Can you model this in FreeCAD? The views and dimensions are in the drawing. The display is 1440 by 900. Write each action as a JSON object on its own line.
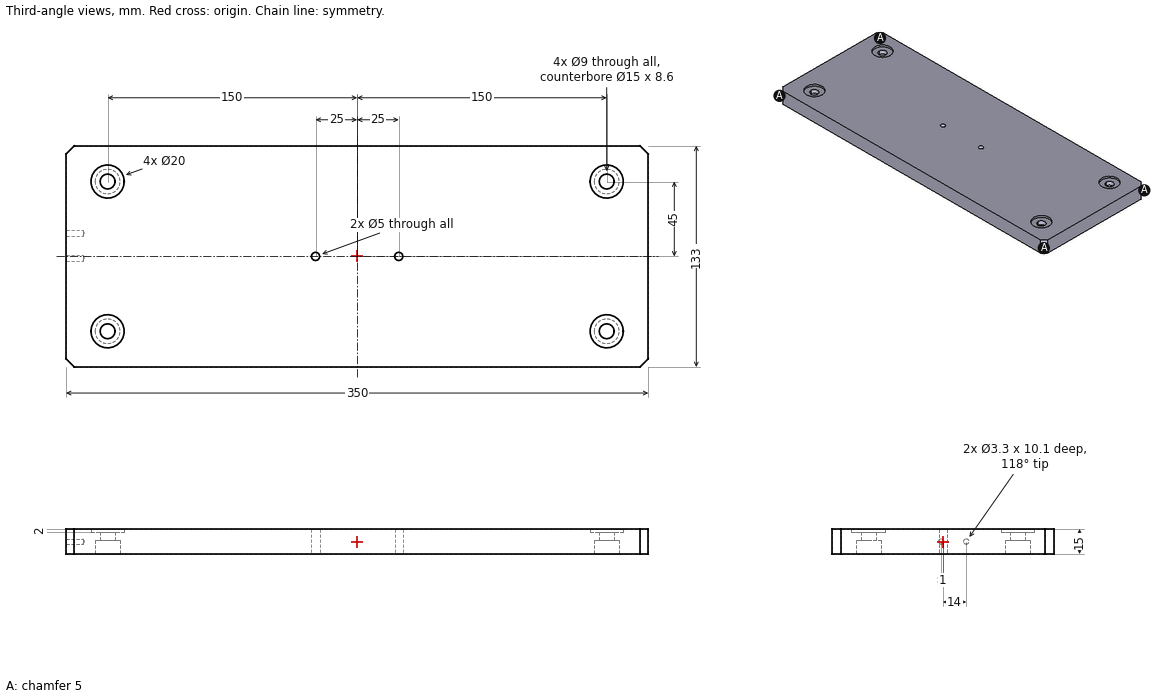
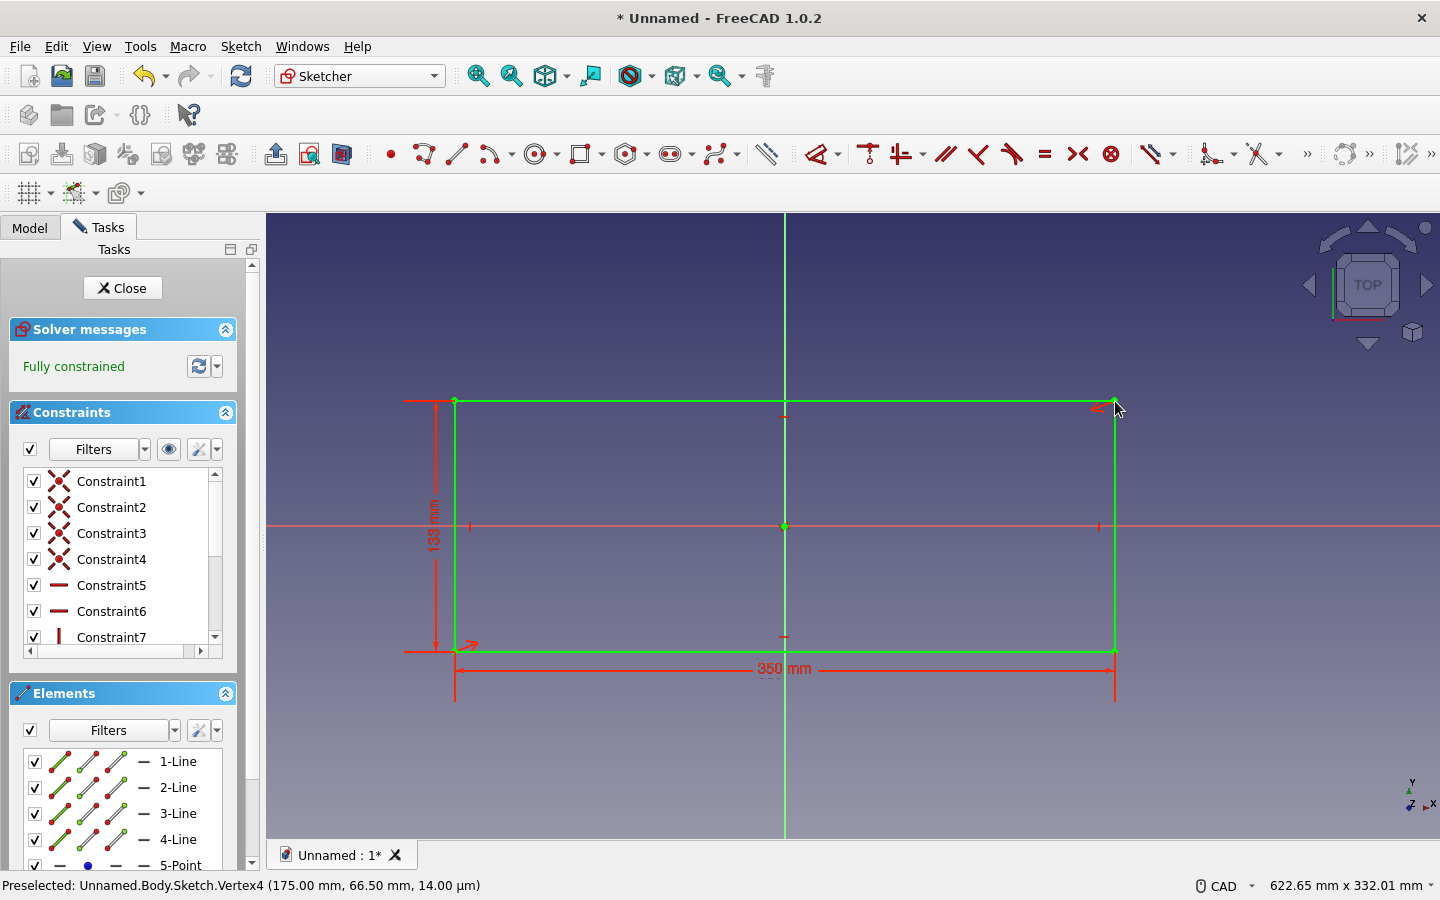
{"action": "left_click", "coordinate": [123, 288]}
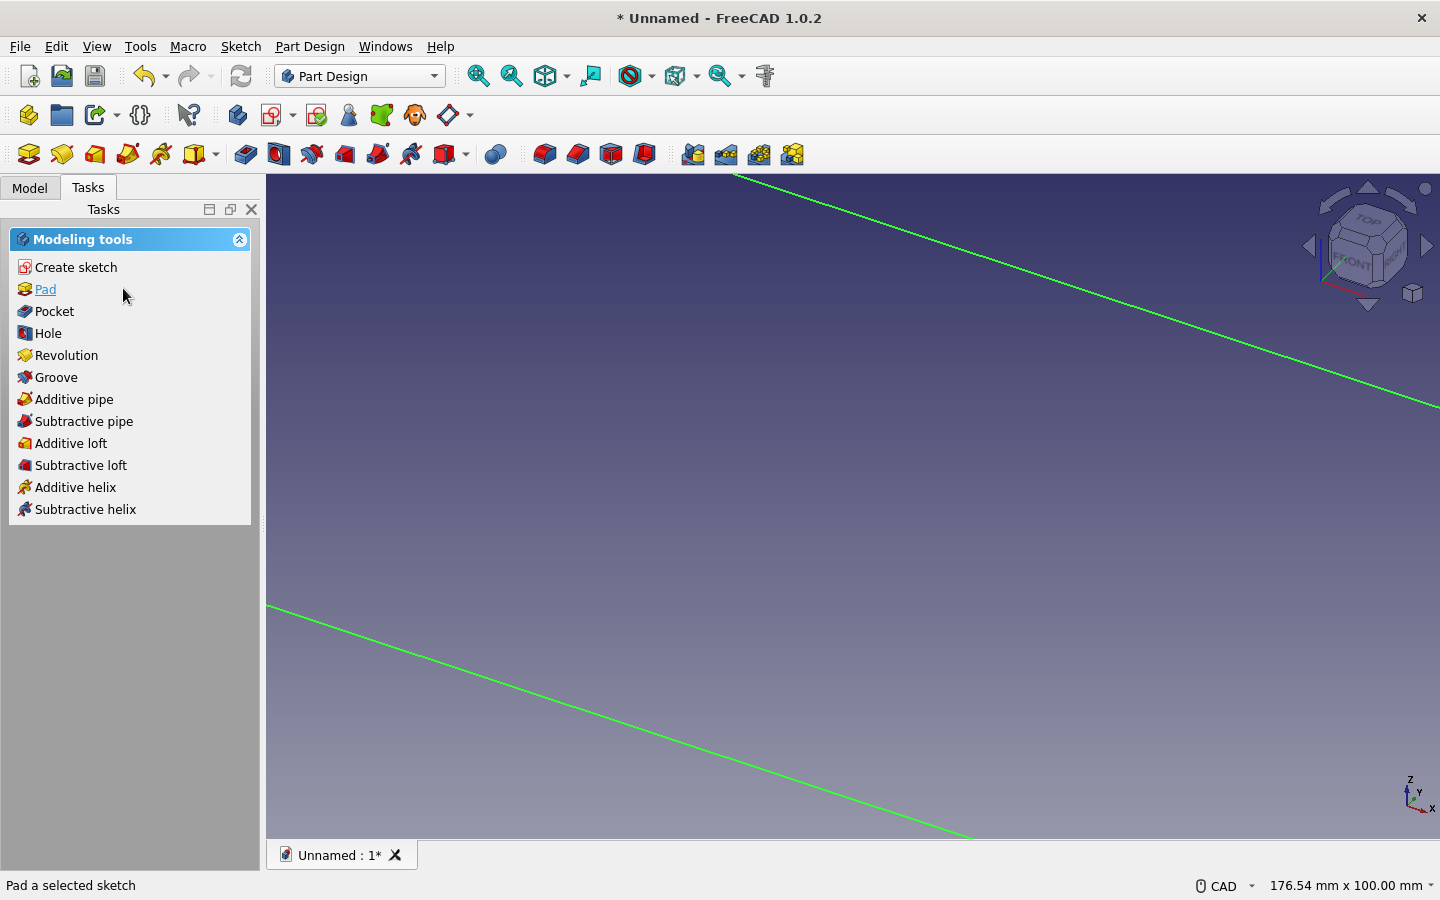
{"action": "left_click", "coordinate": [29, 154]}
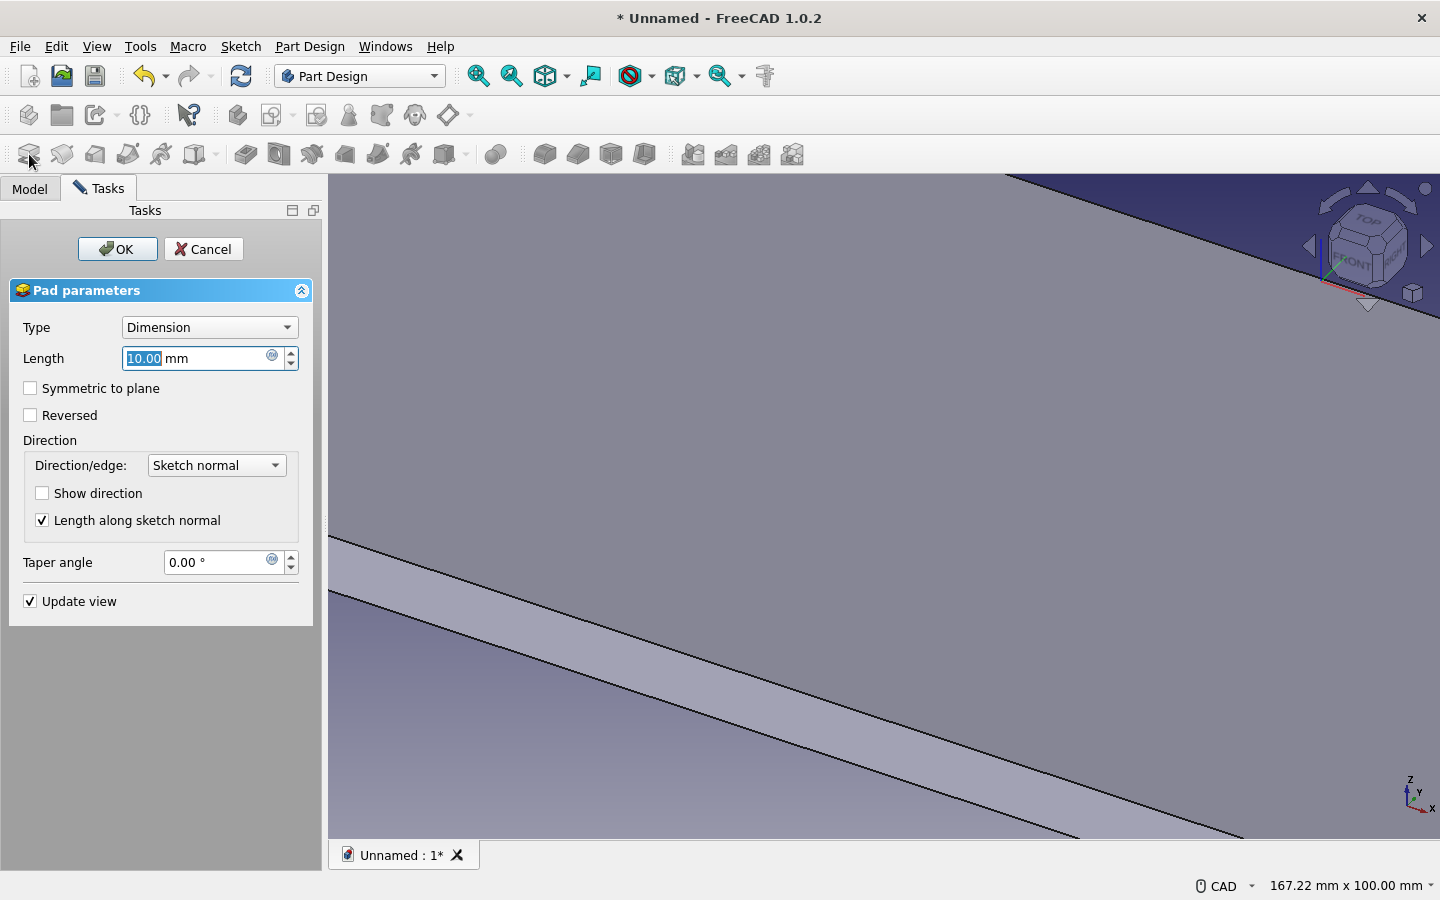
{"action": "type", "text": "15"}
{"action": "key", "text": "Tab"}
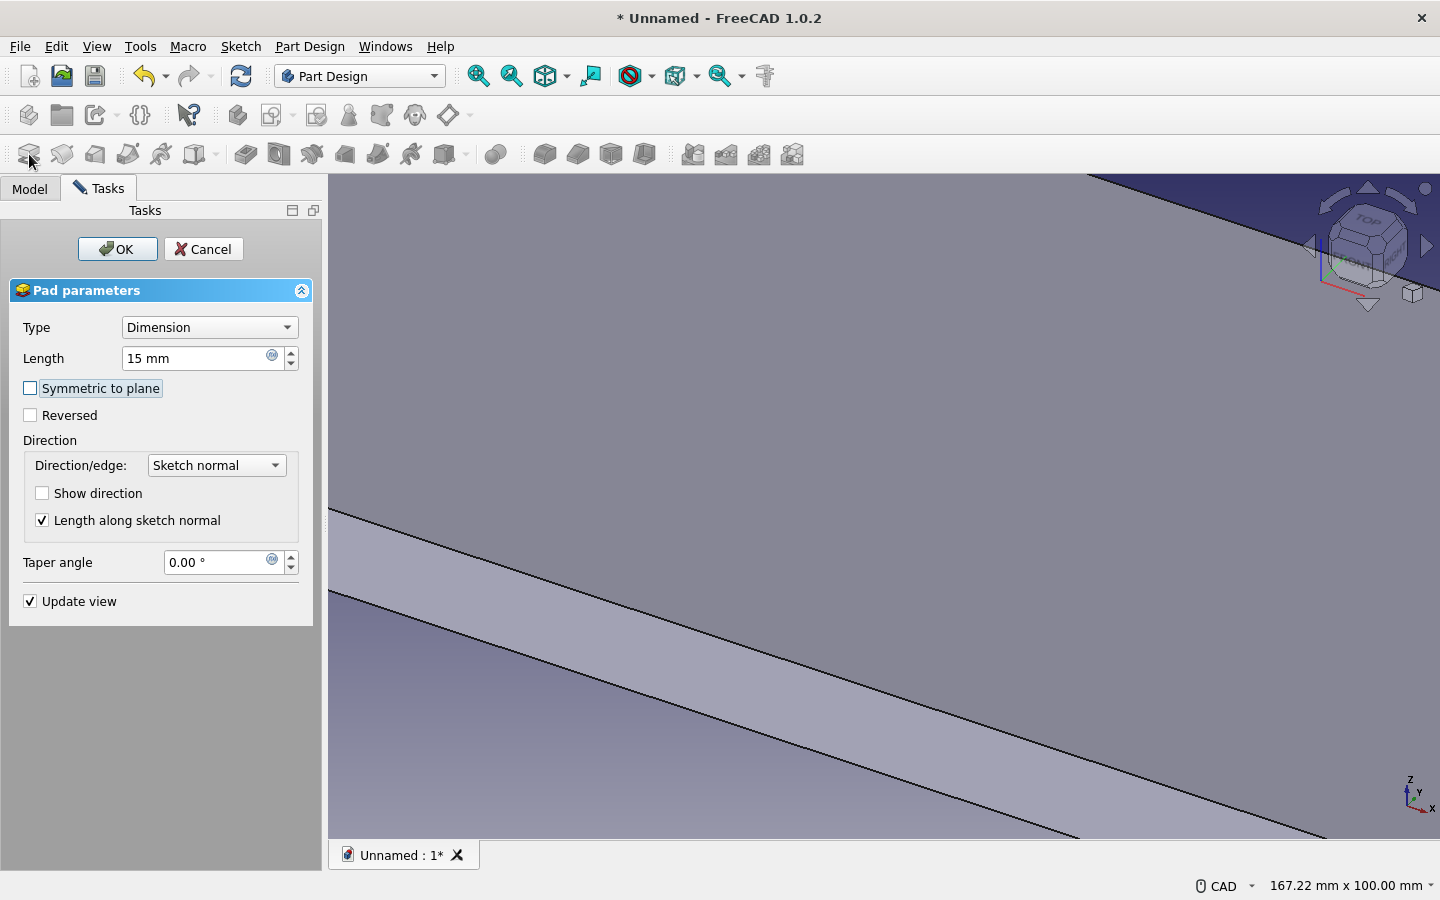
{"action": "left_click", "coordinate": [31, 388]}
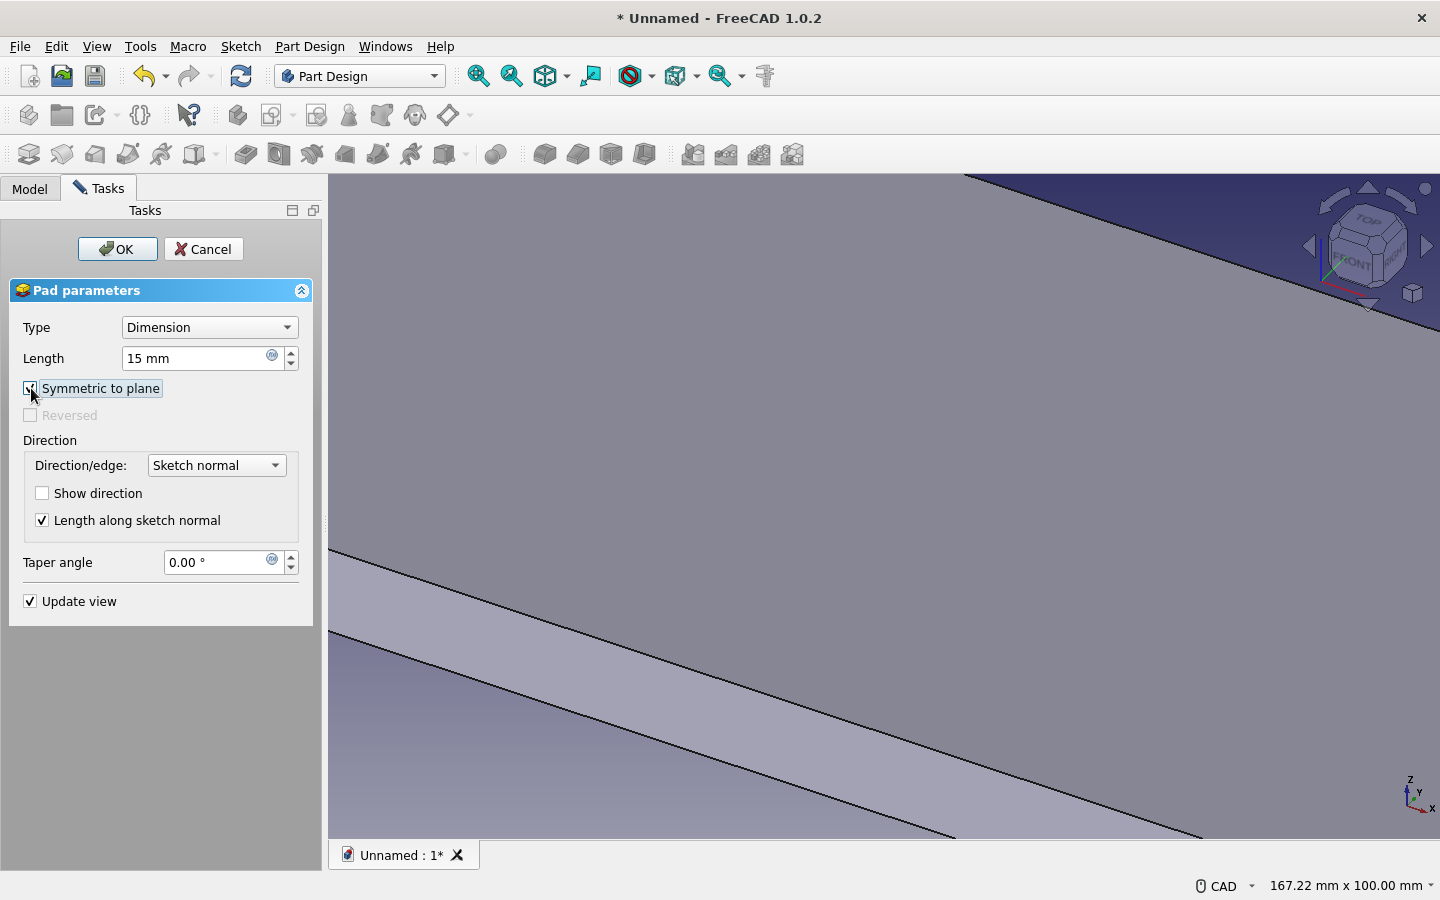
{"action": "left_click", "coordinate": [118, 249]}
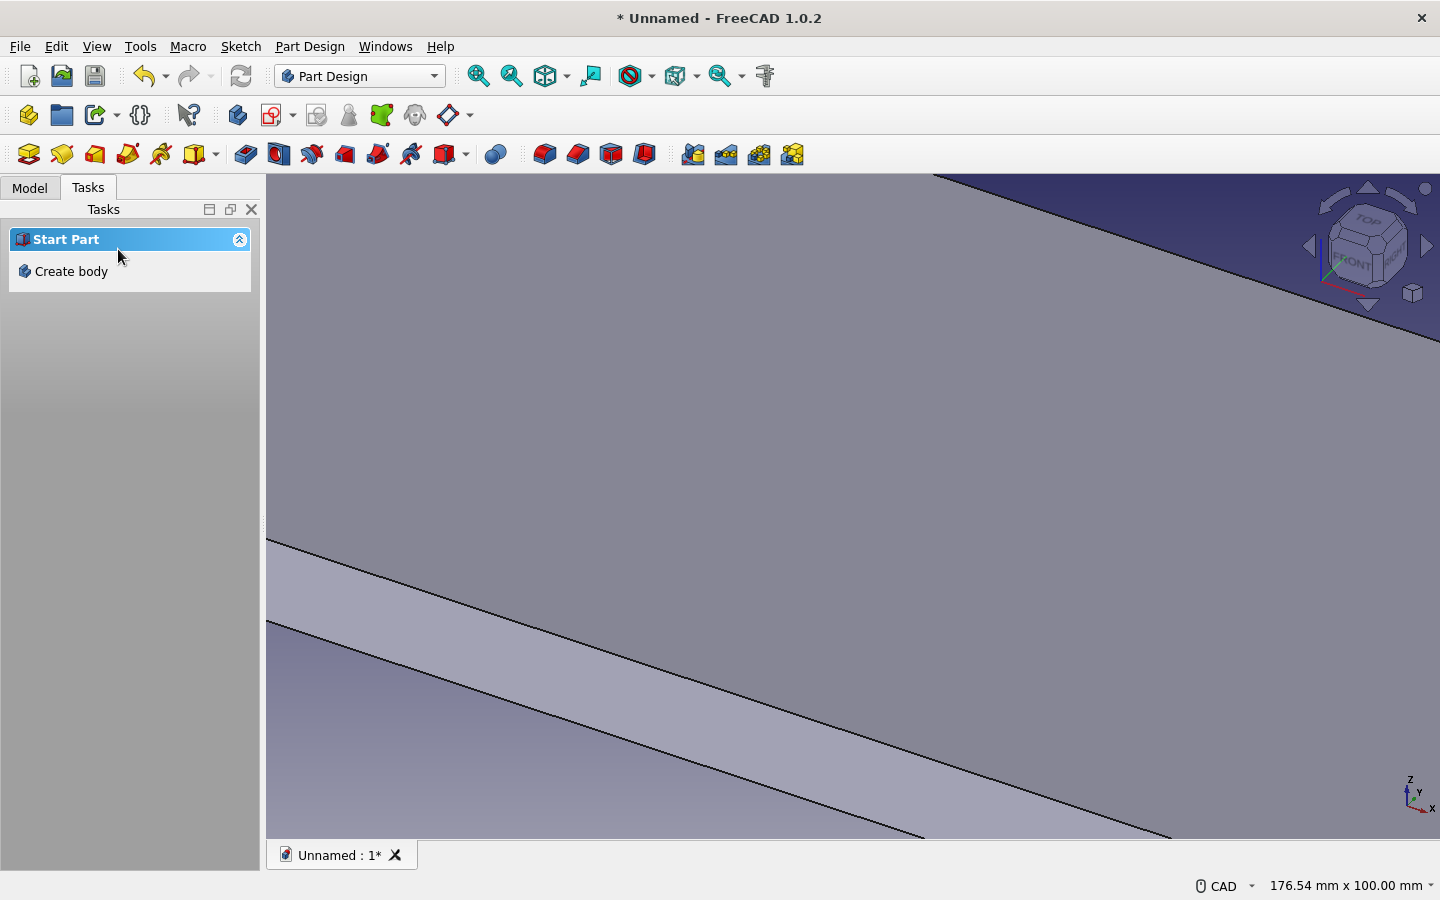
{"action": "left_click", "coordinate": [479, 76]}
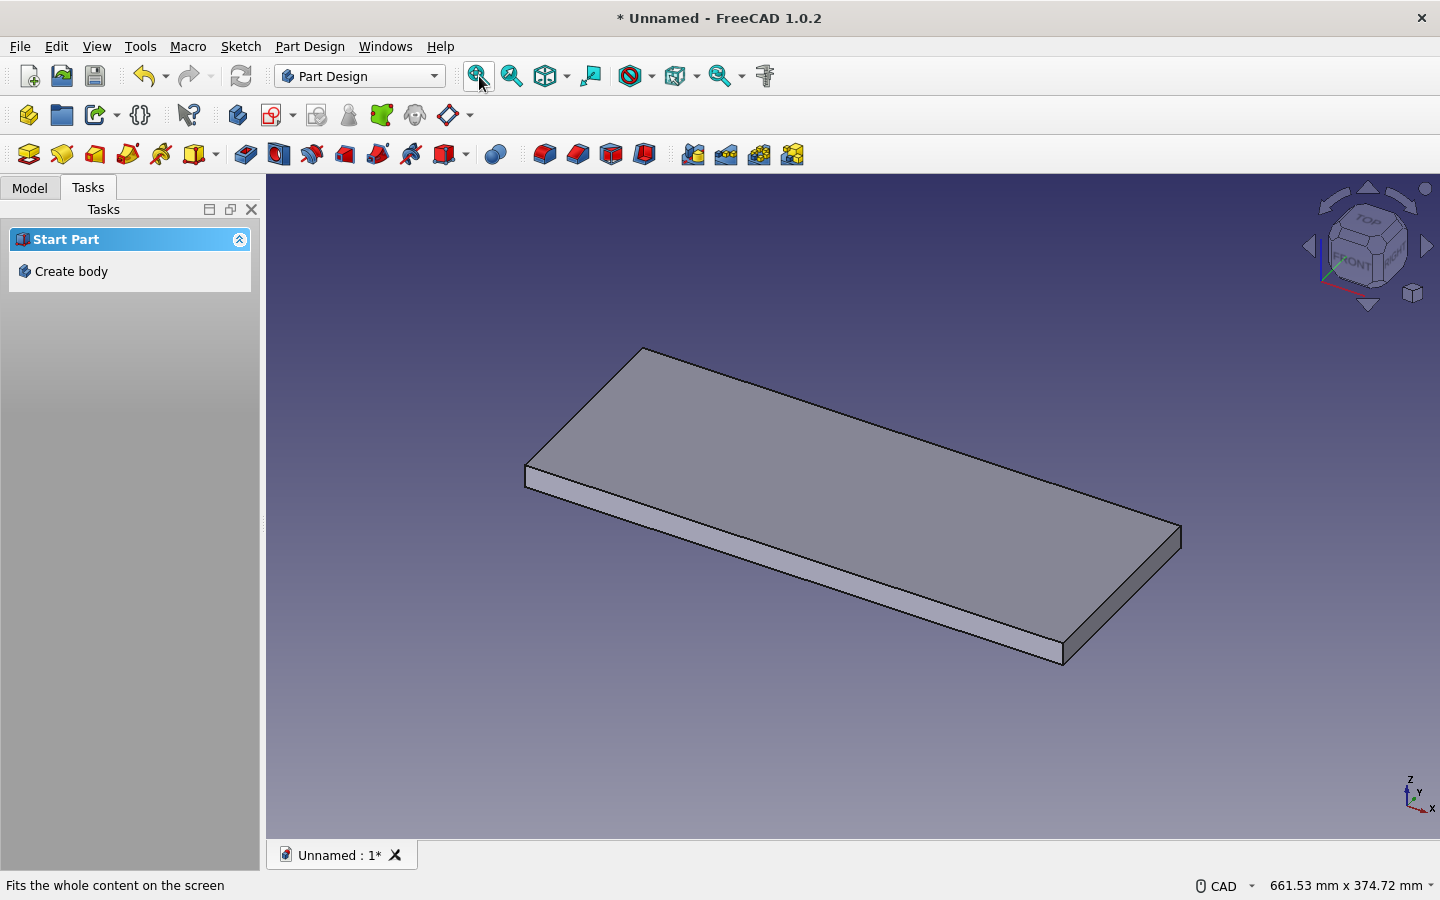
{"action": "key", "text": "5"}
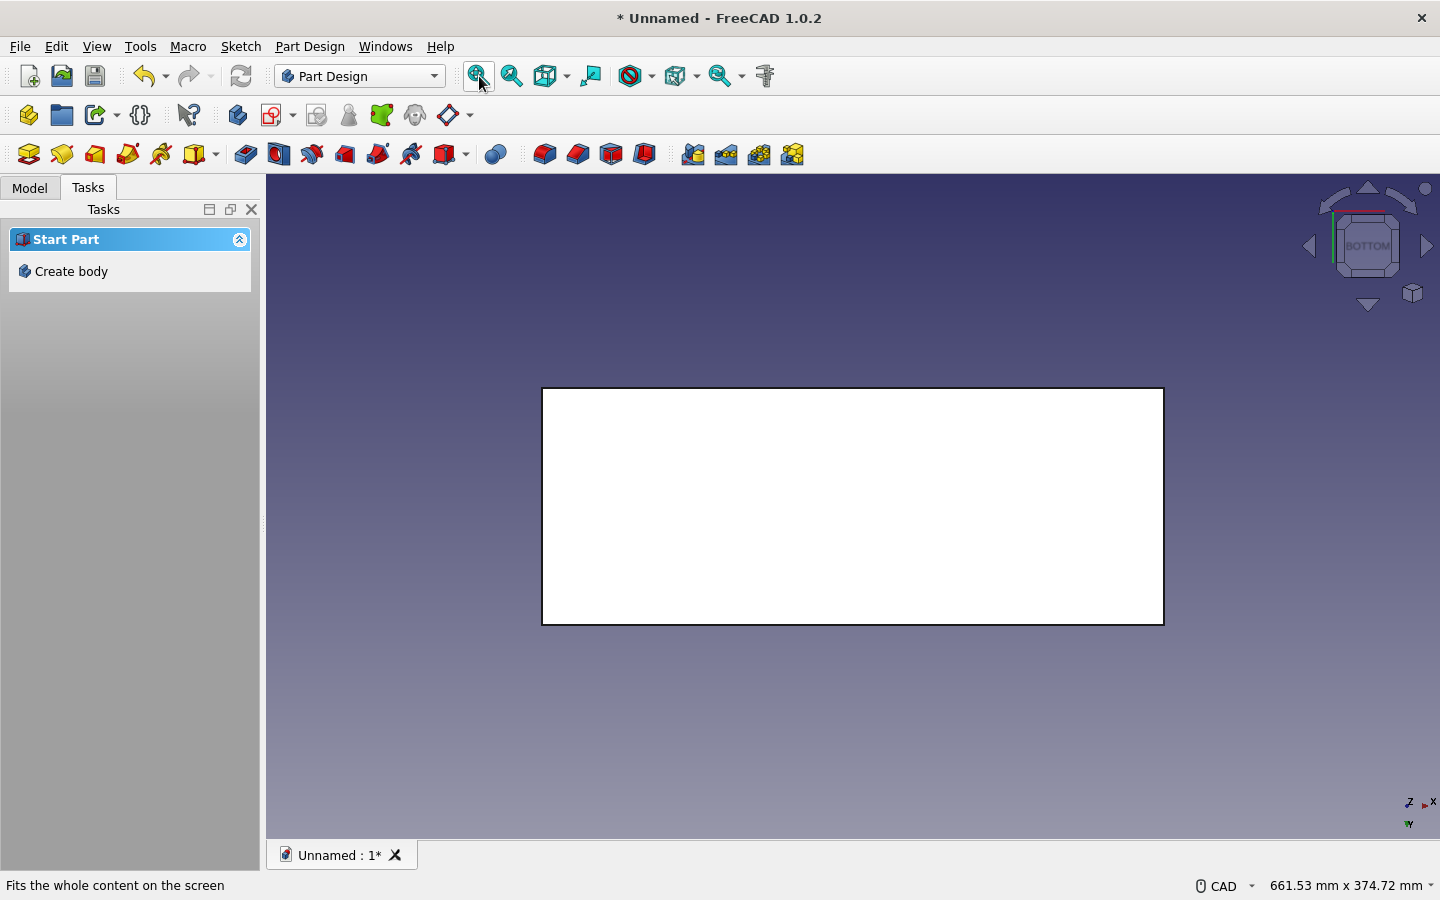
{"action": "left_click", "coordinate": [1030, 505]}